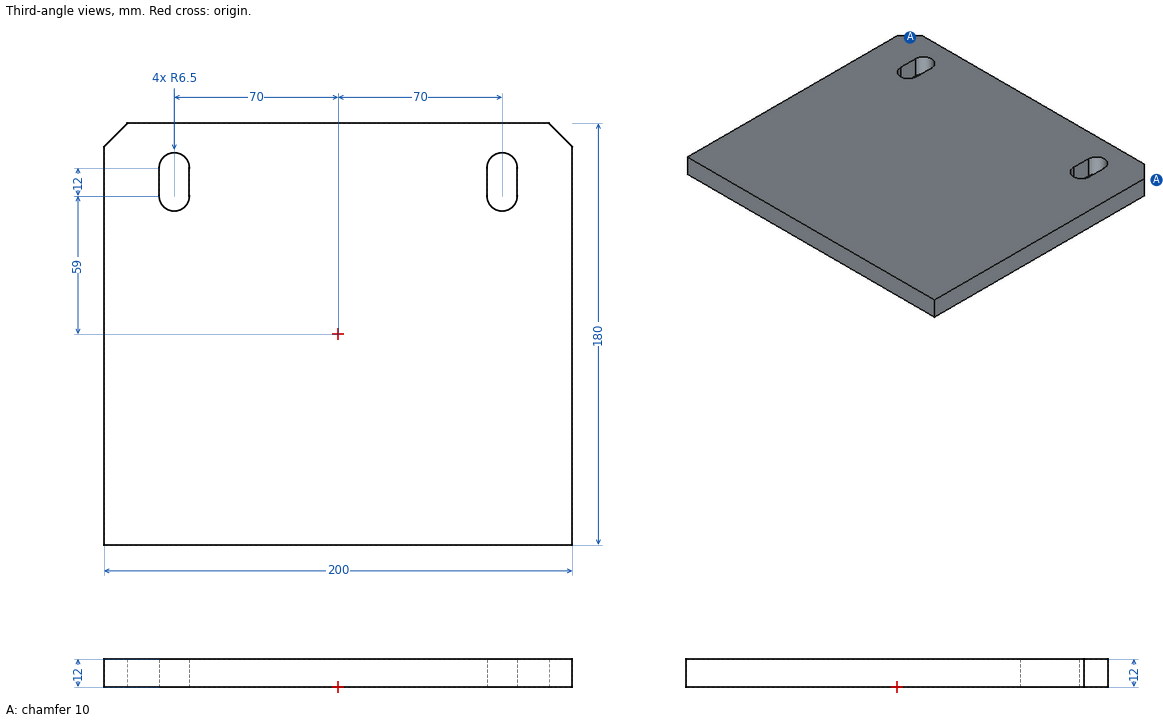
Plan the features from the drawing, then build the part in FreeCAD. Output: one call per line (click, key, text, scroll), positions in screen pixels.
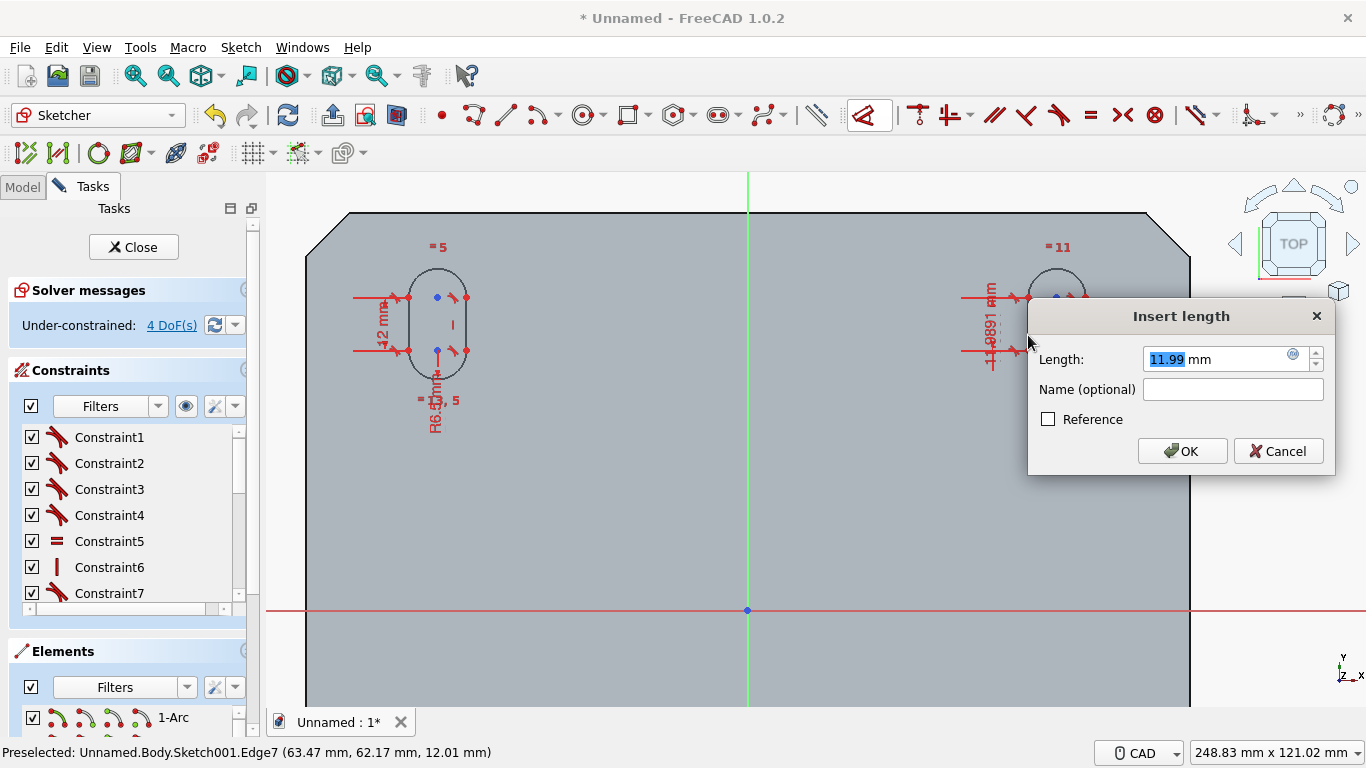
text(12)
key(Return)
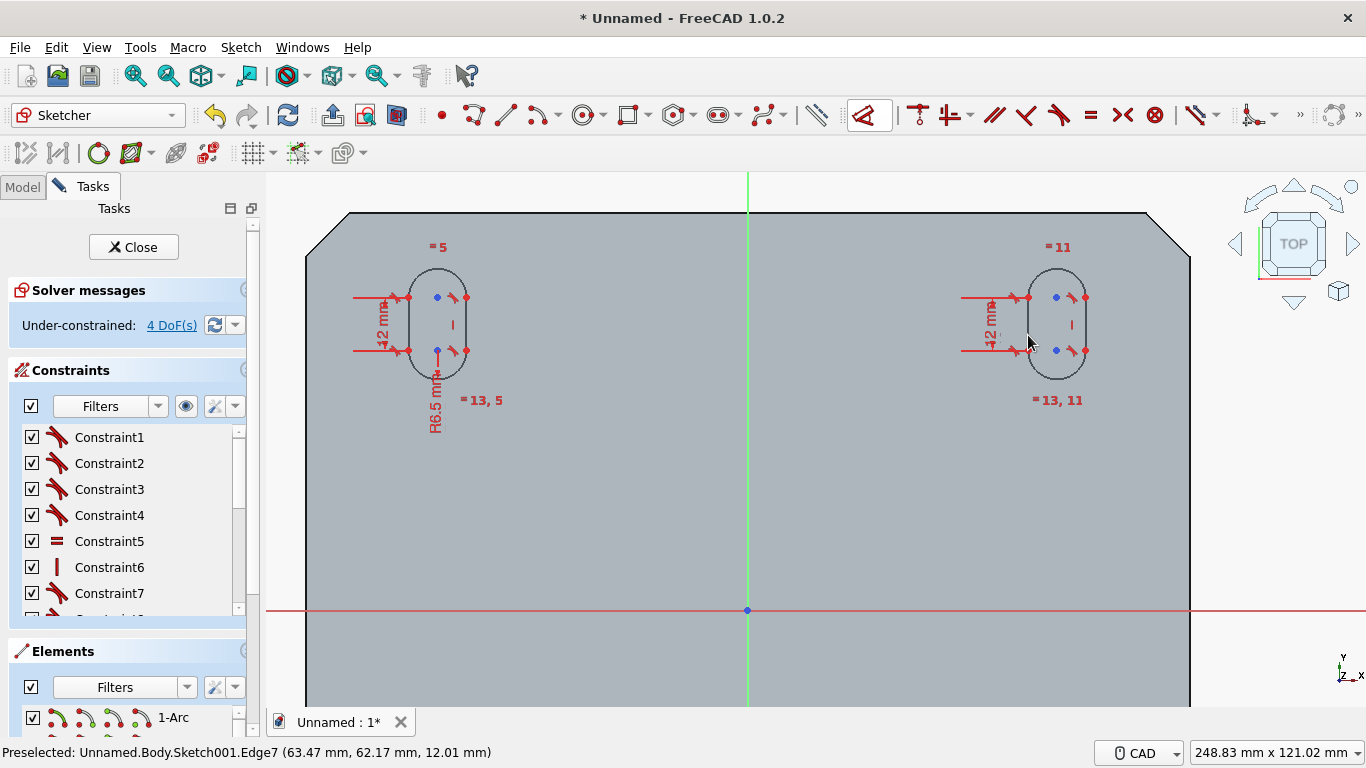
click(409, 351)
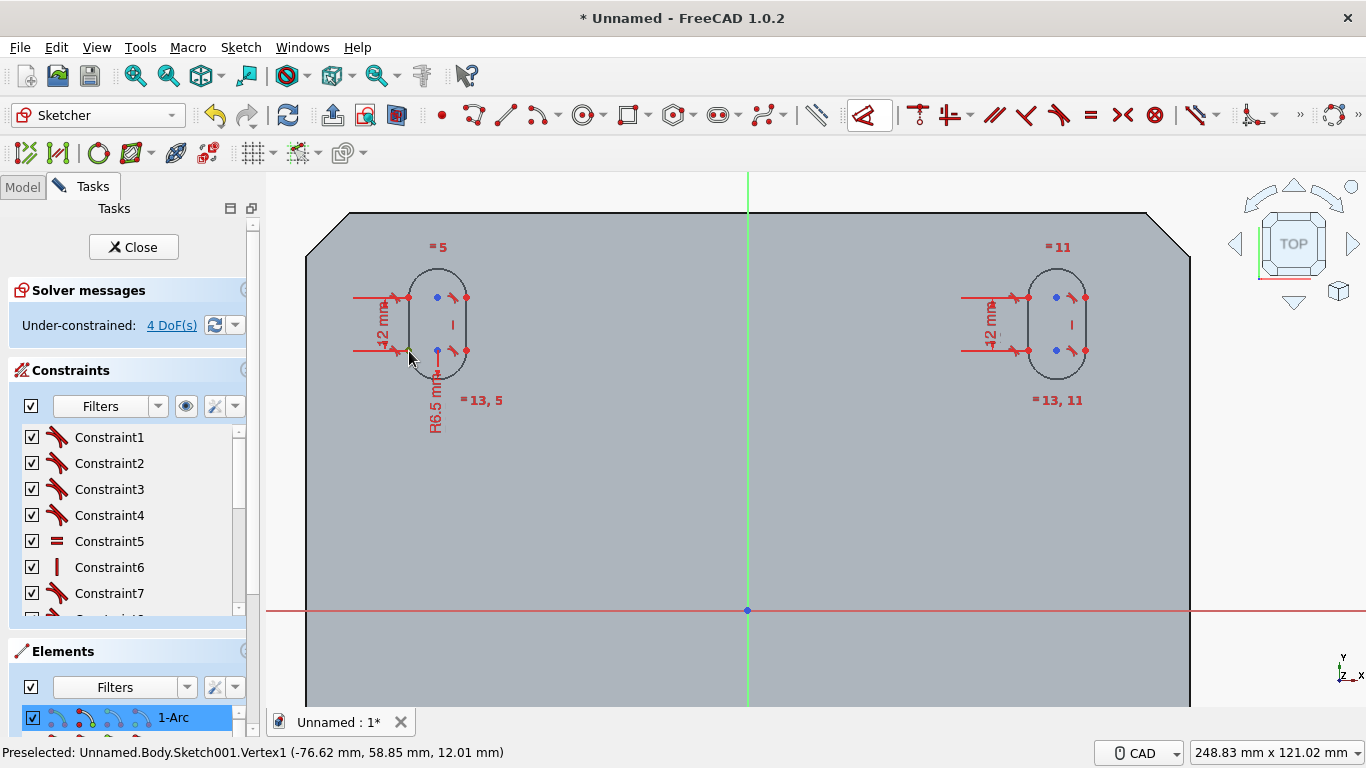
click(886, 116)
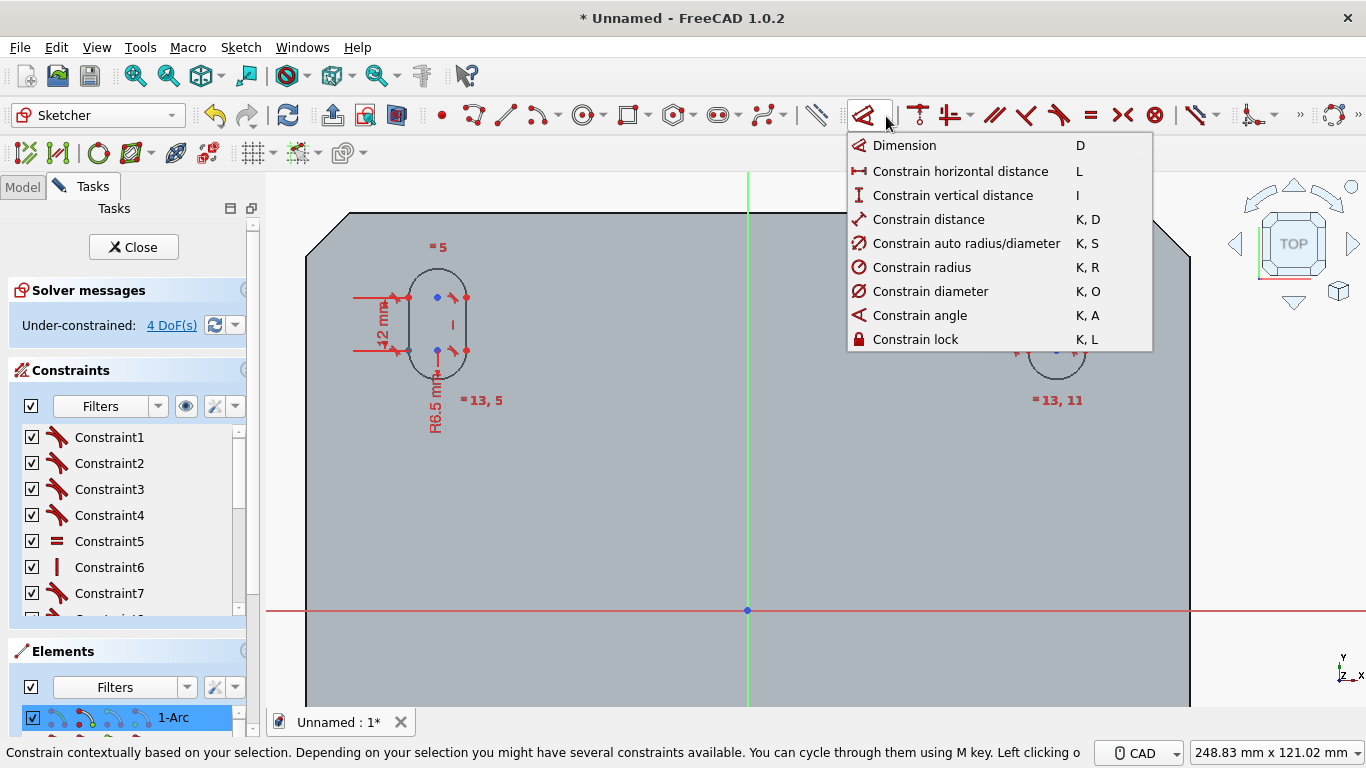
click(1000, 195)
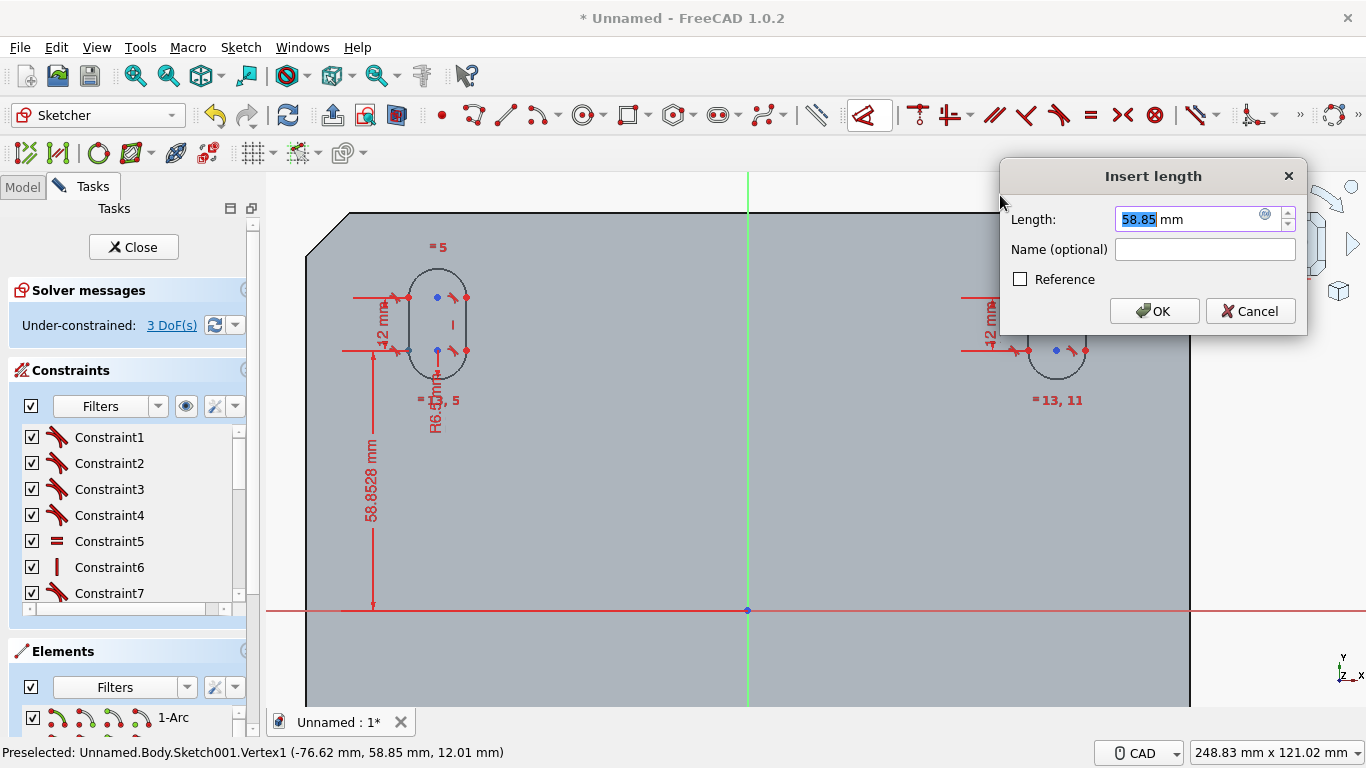
text(59)
key(Return)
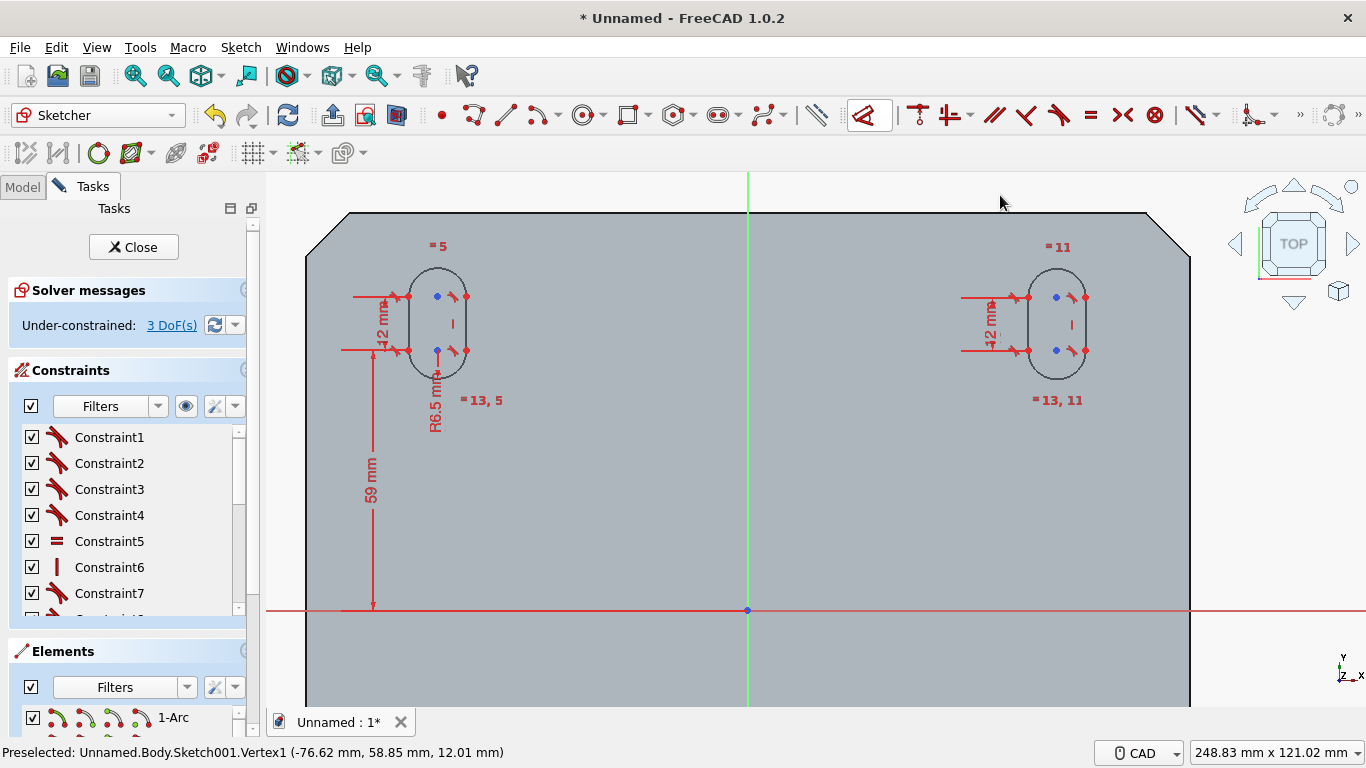
click(1028, 351)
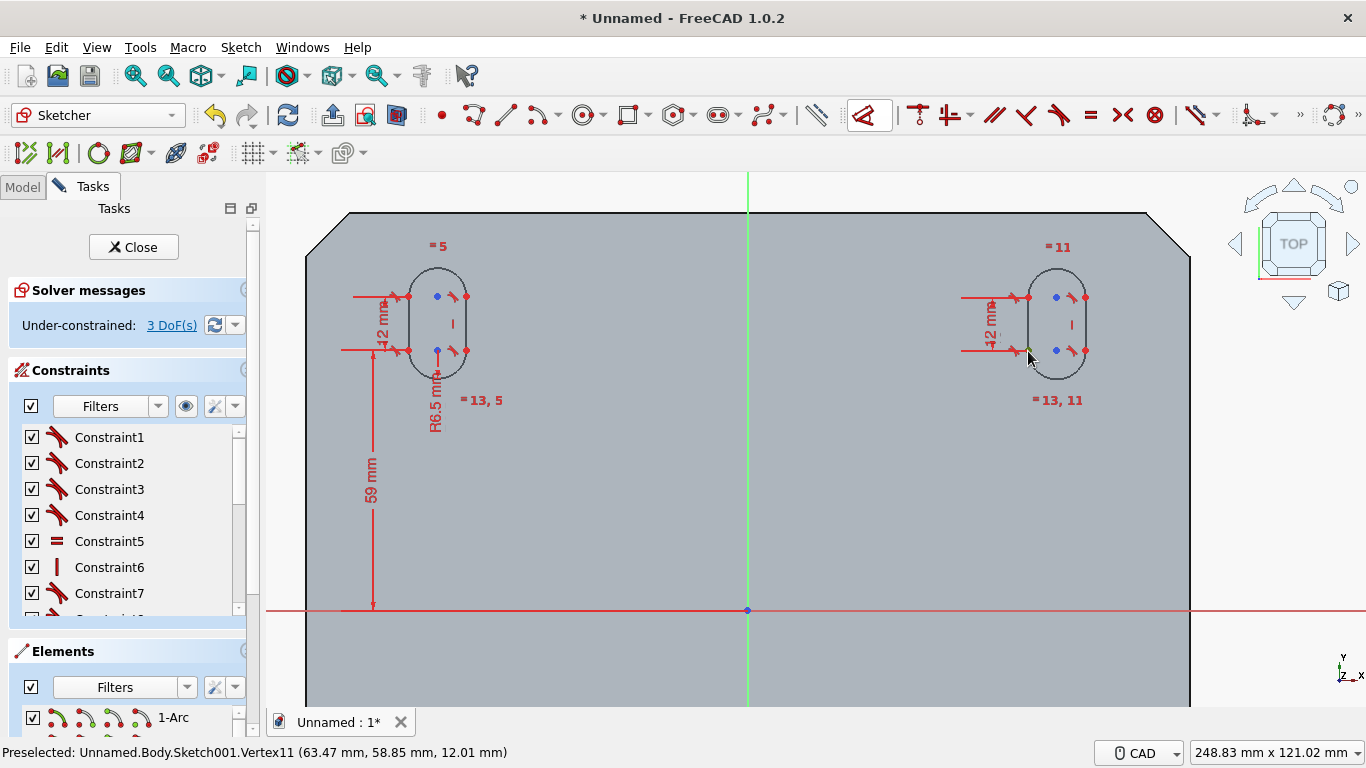
key(i)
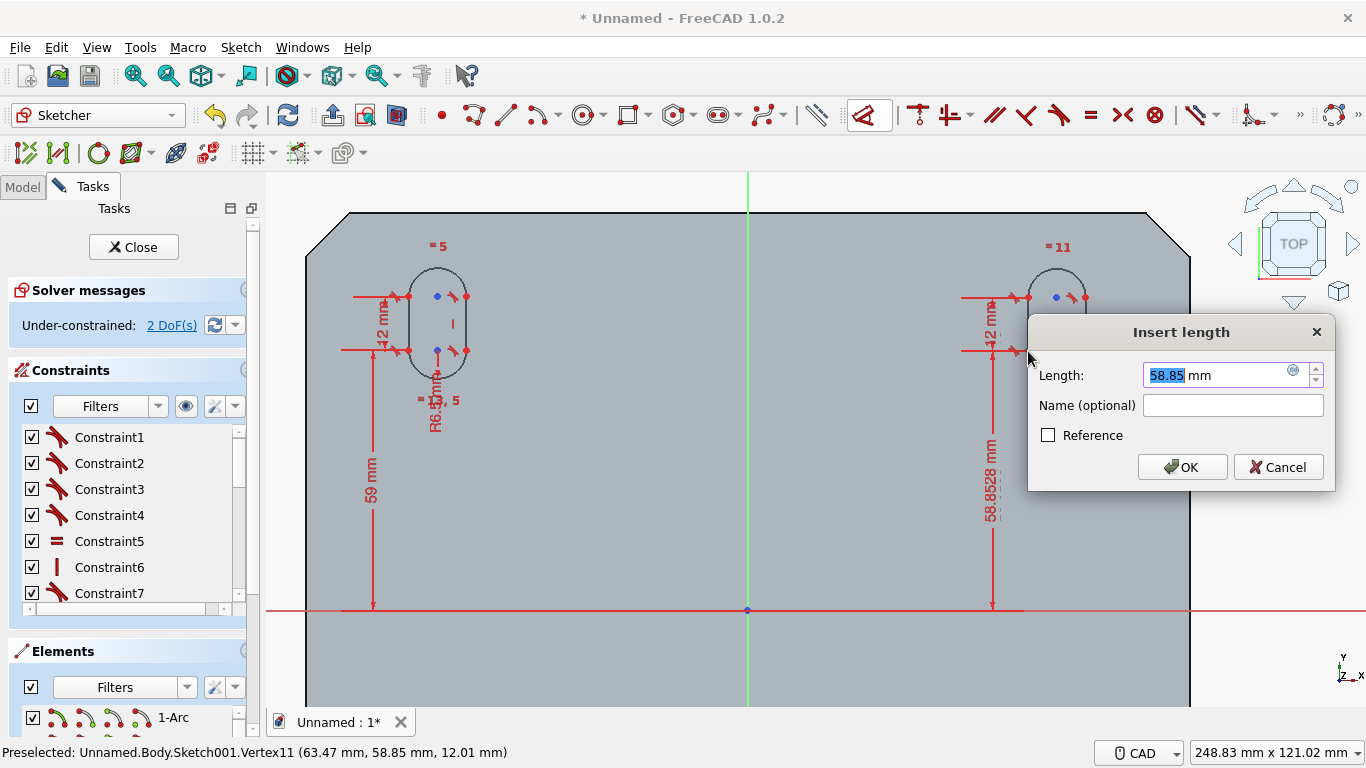
text(59)
key(Return)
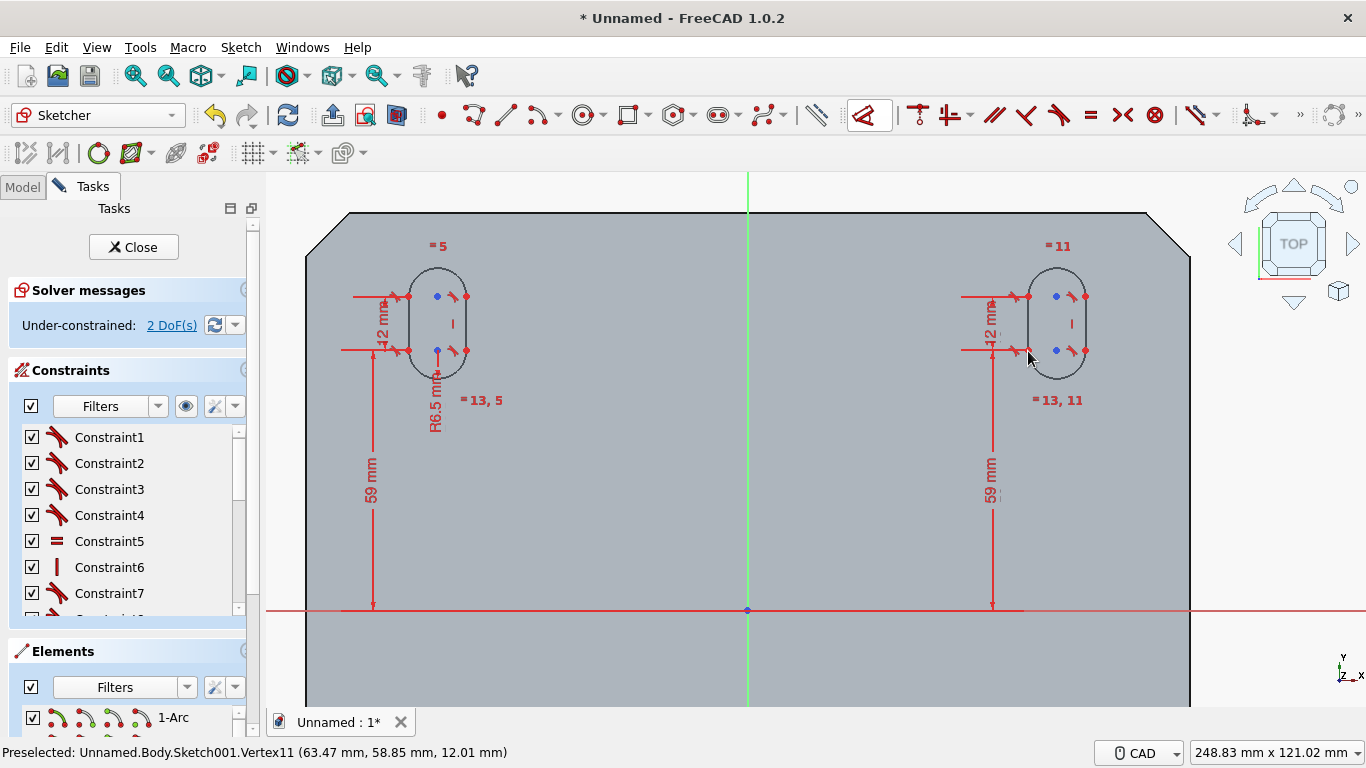
click(438, 350)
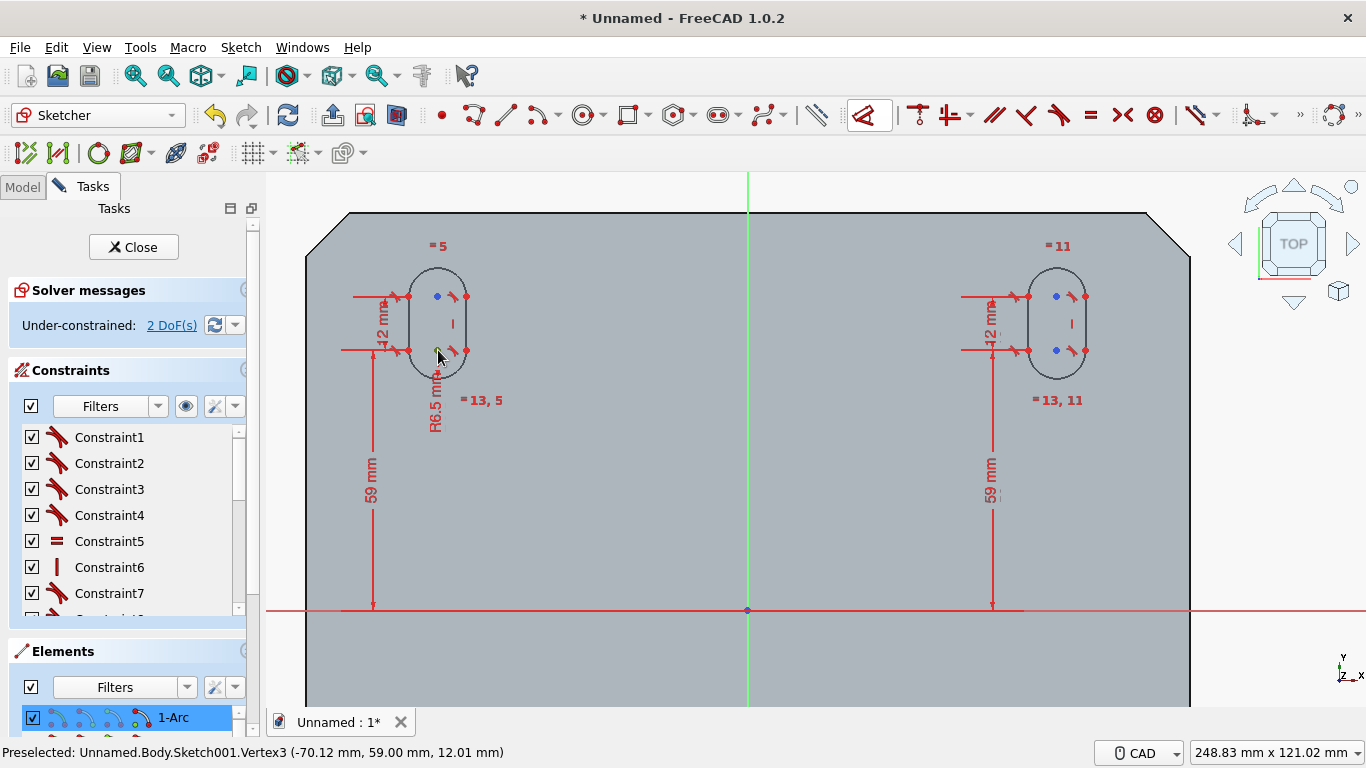
key(l)